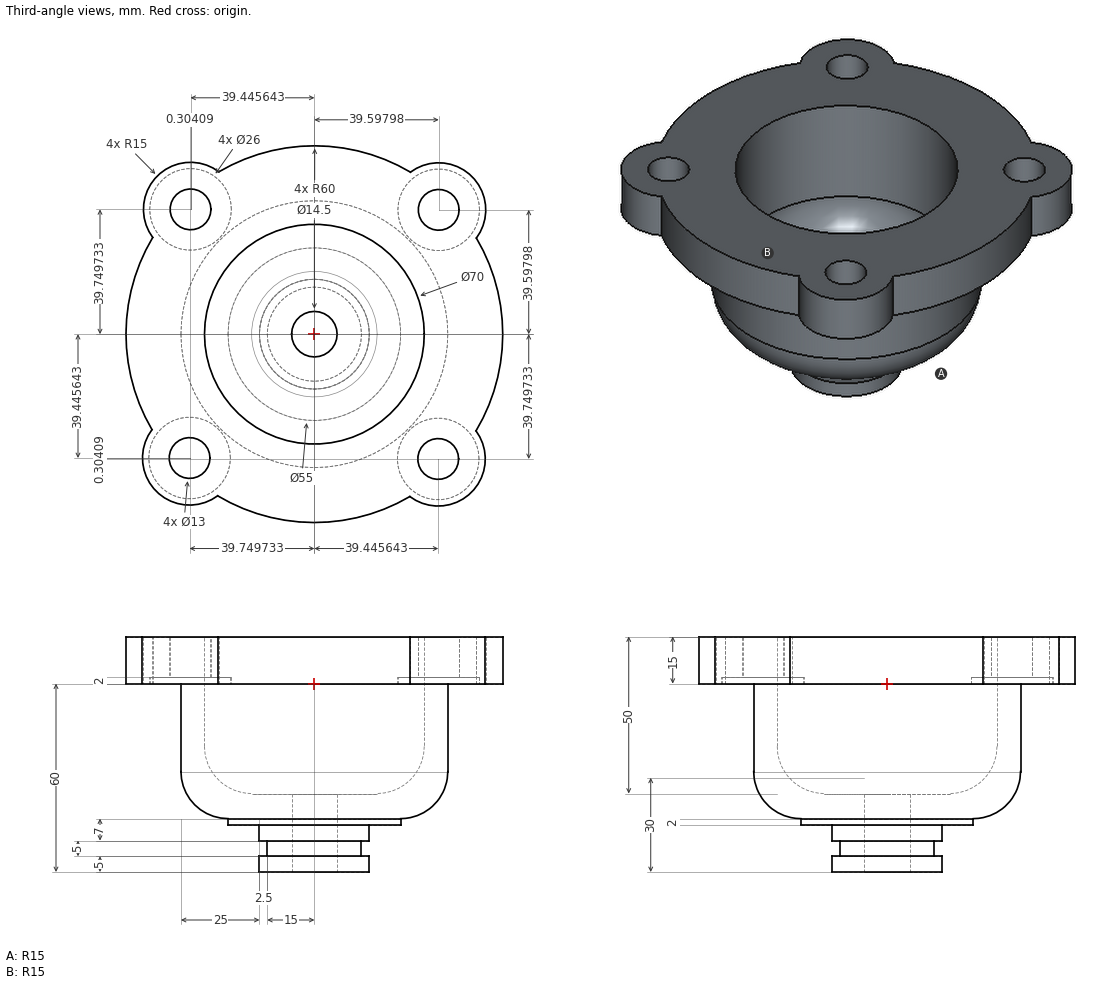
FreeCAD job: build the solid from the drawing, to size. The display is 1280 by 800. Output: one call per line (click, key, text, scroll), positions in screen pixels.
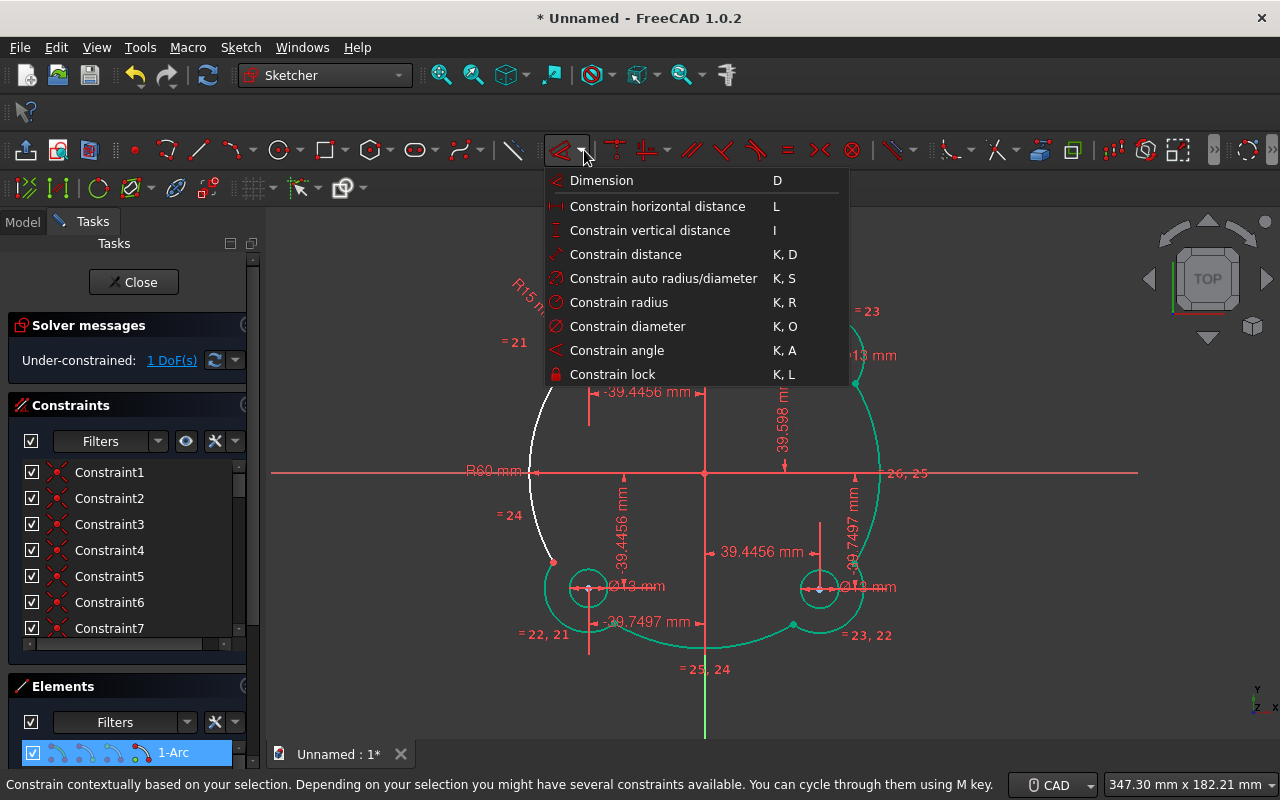
click(697, 230)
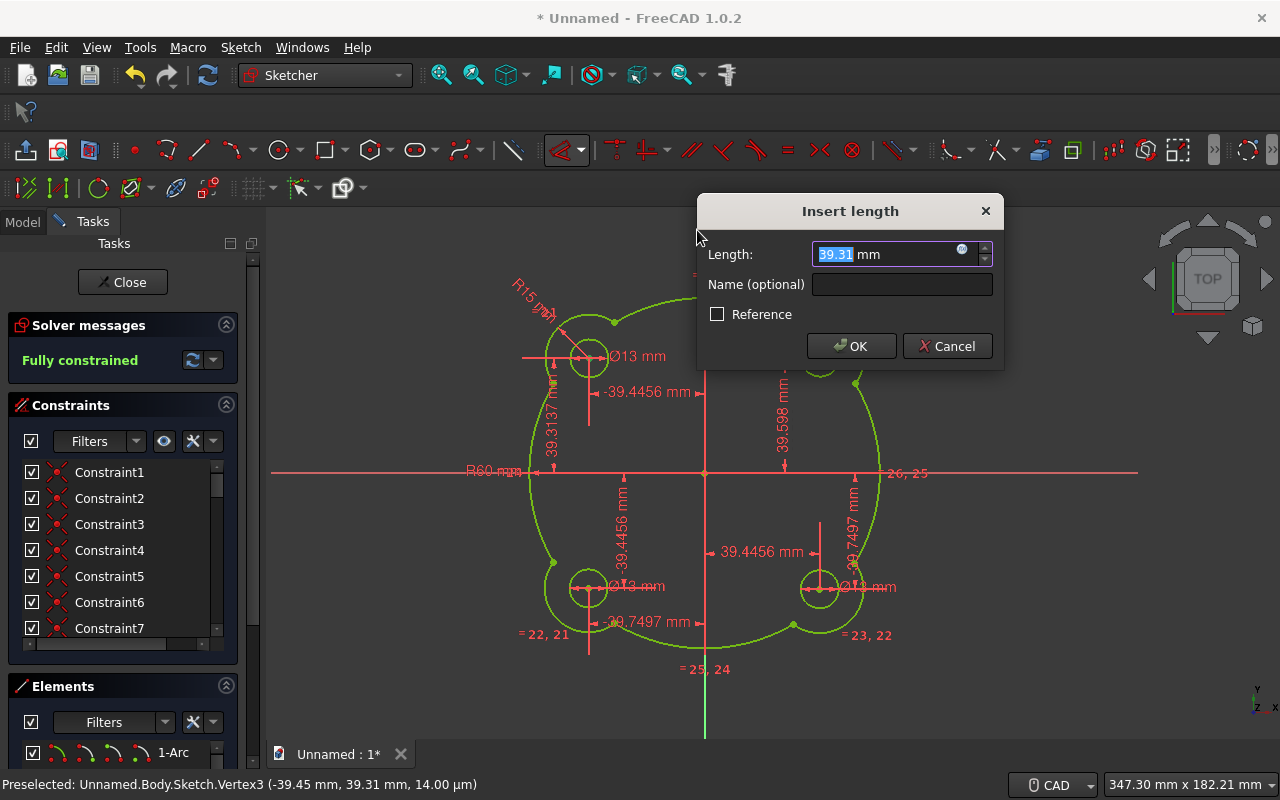
text(39.749733)
key(Return)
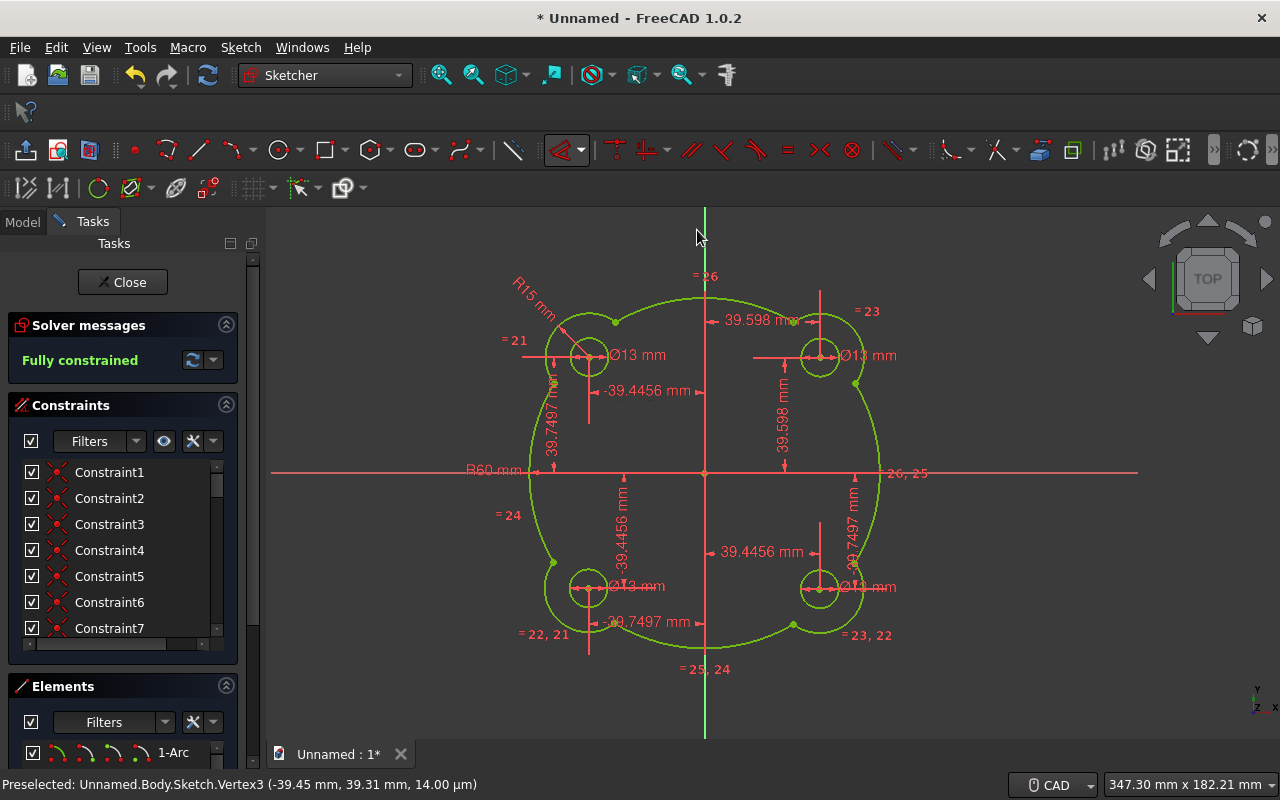
click(123, 282)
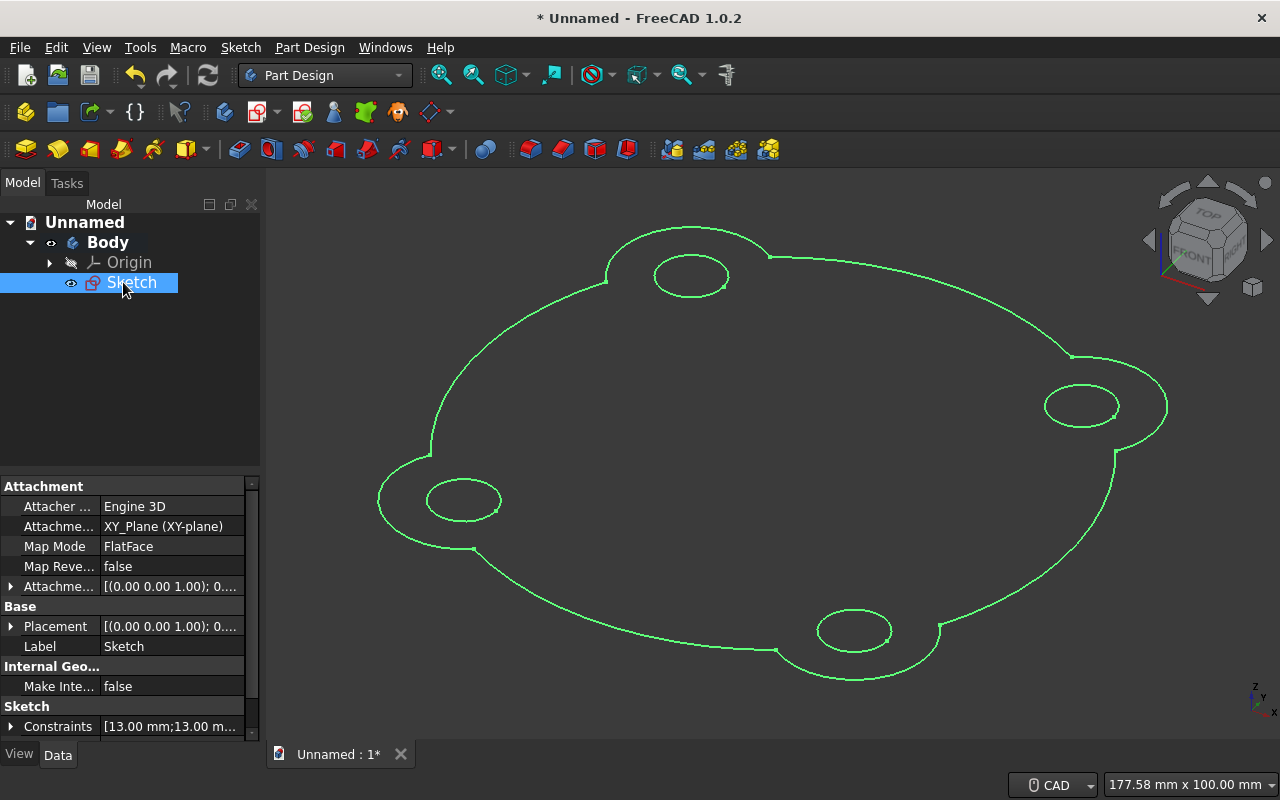
click(26, 150)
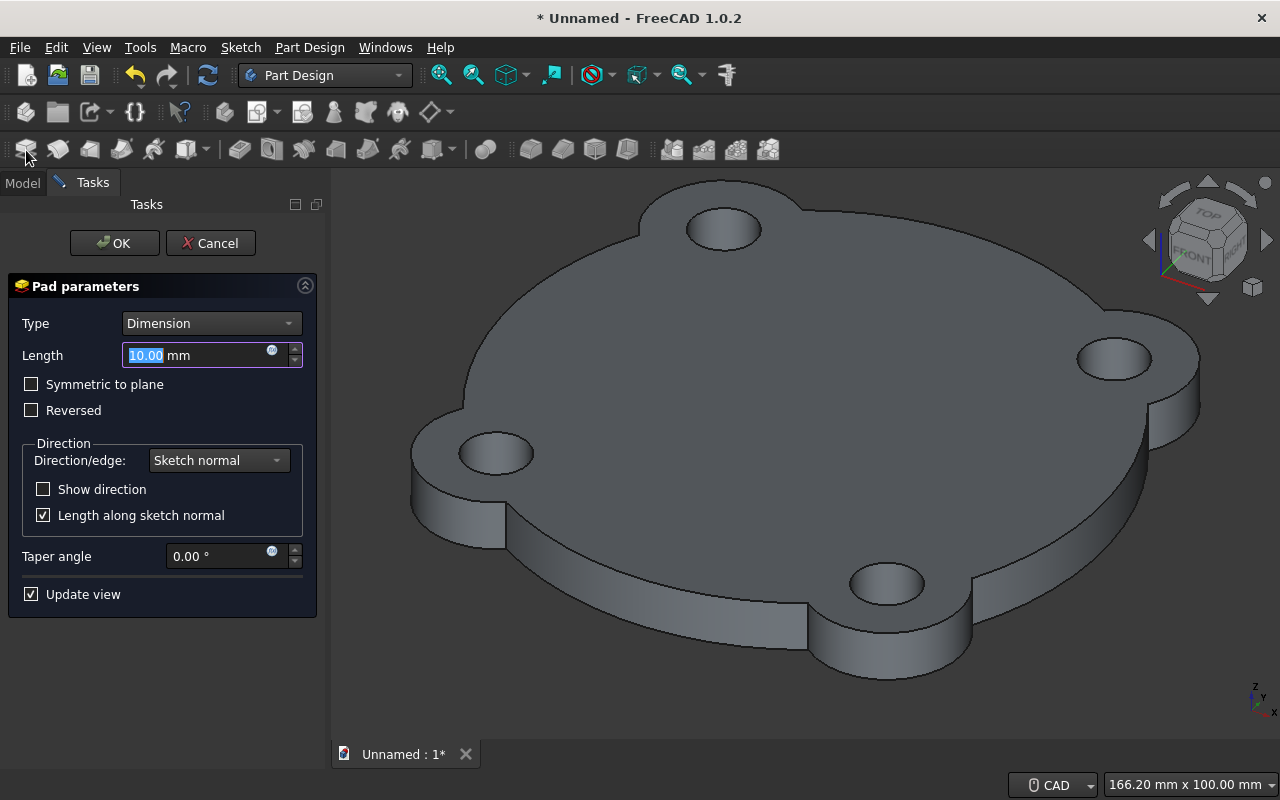
text(15)
key(Tab)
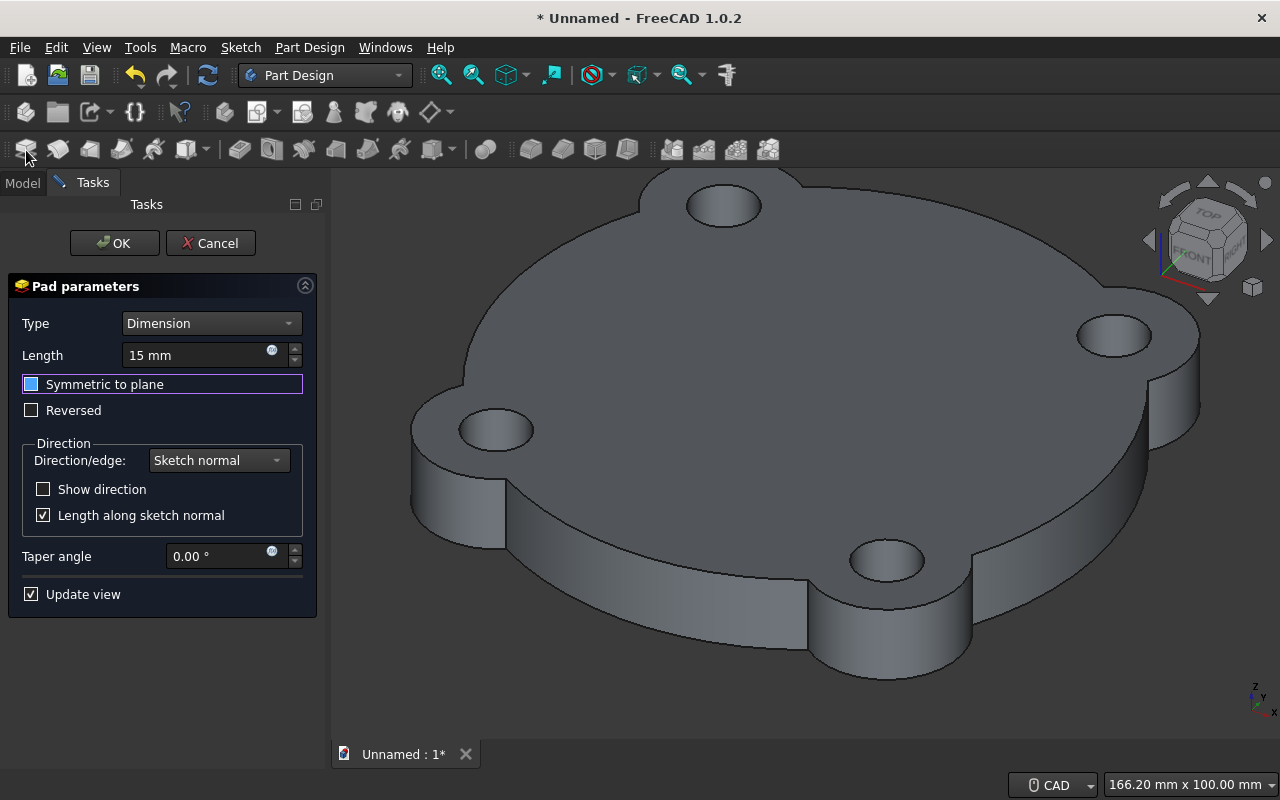
click(115, 243)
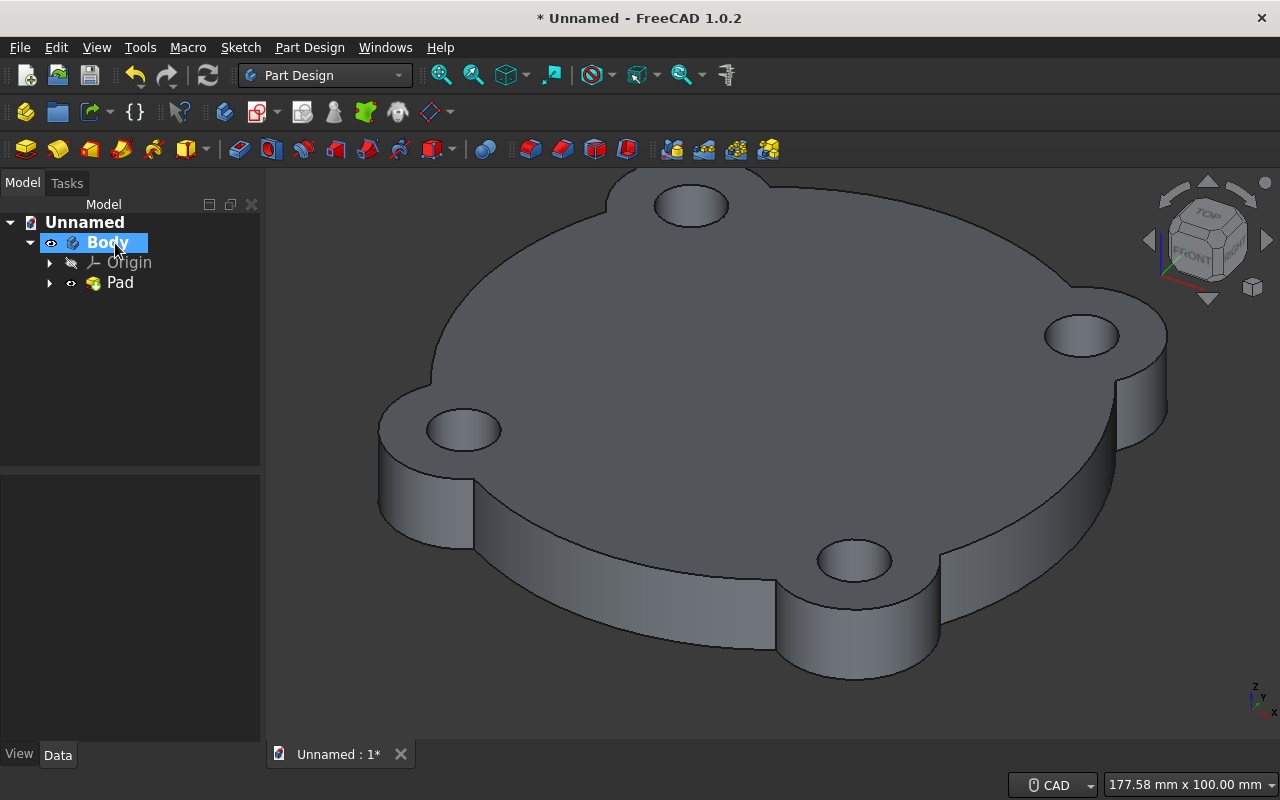
click(442, 76)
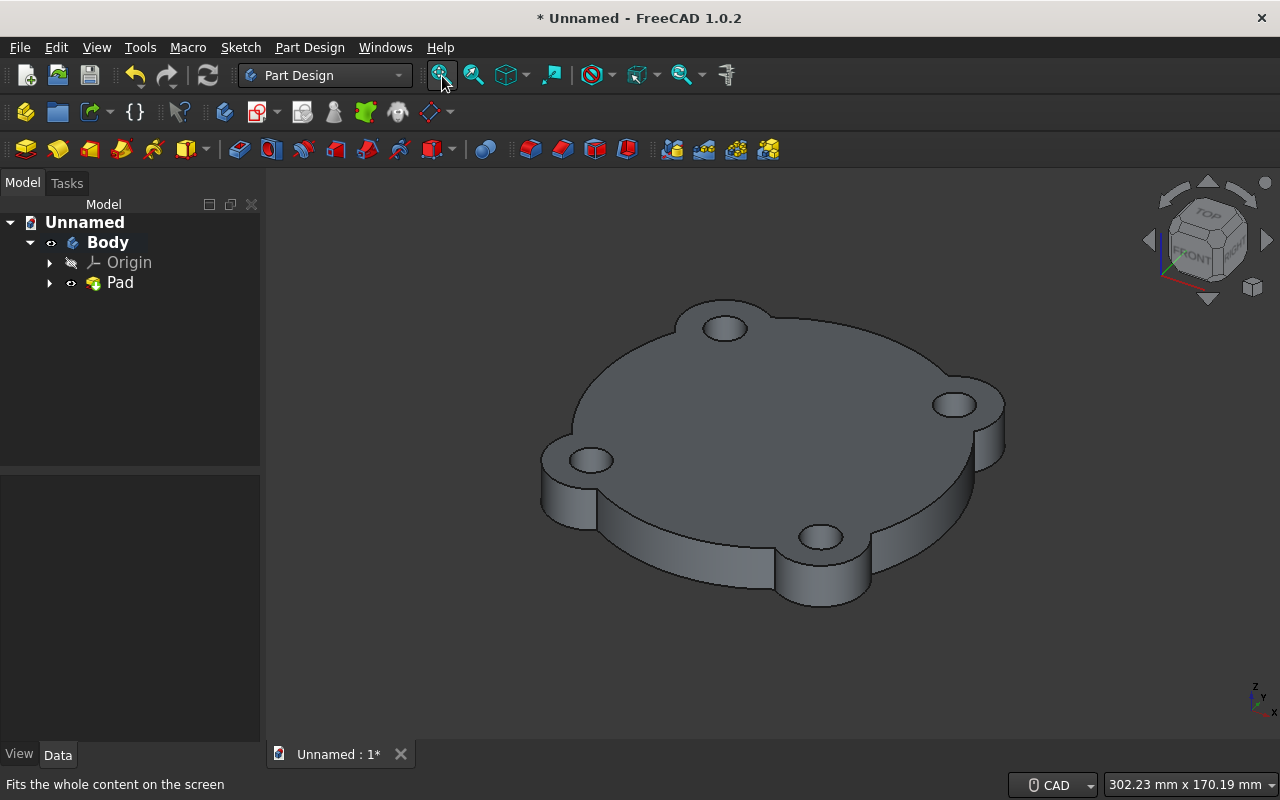
click(50, 263)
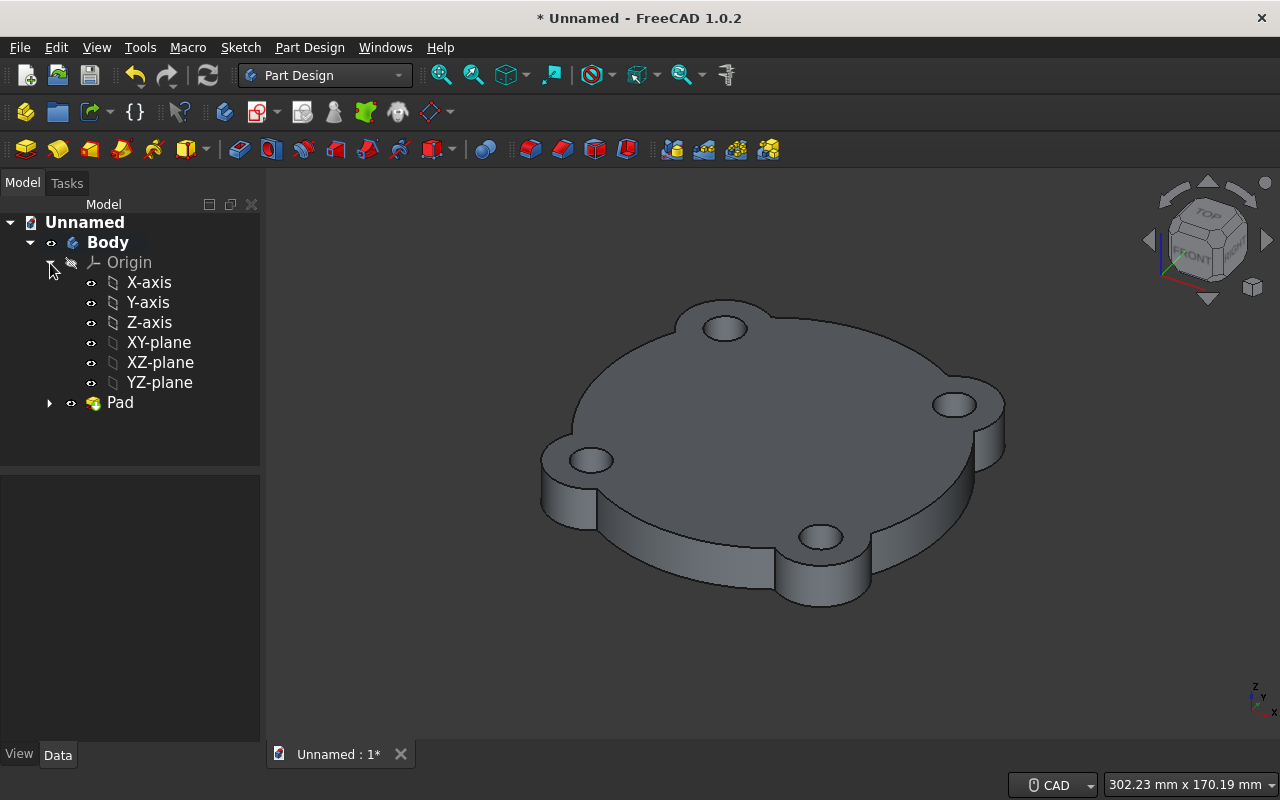
click(136, 343)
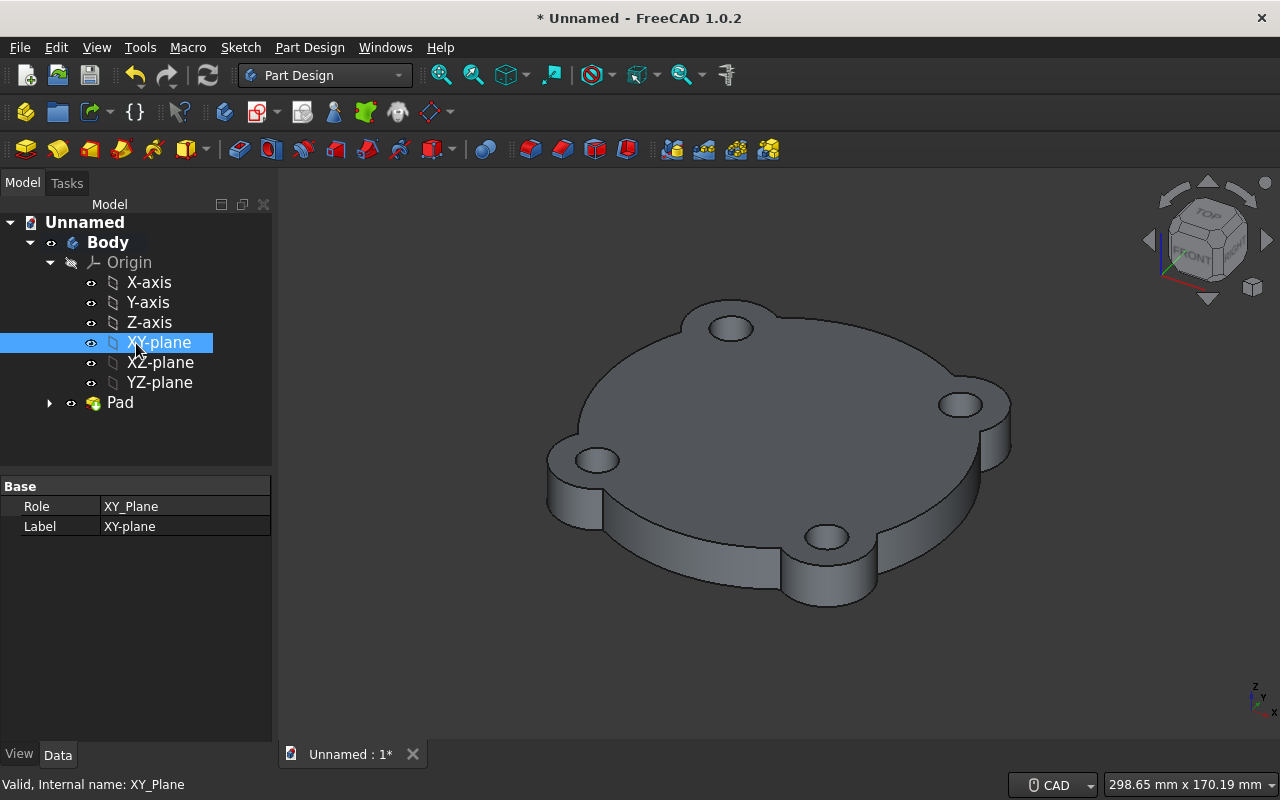
click(430, 112)